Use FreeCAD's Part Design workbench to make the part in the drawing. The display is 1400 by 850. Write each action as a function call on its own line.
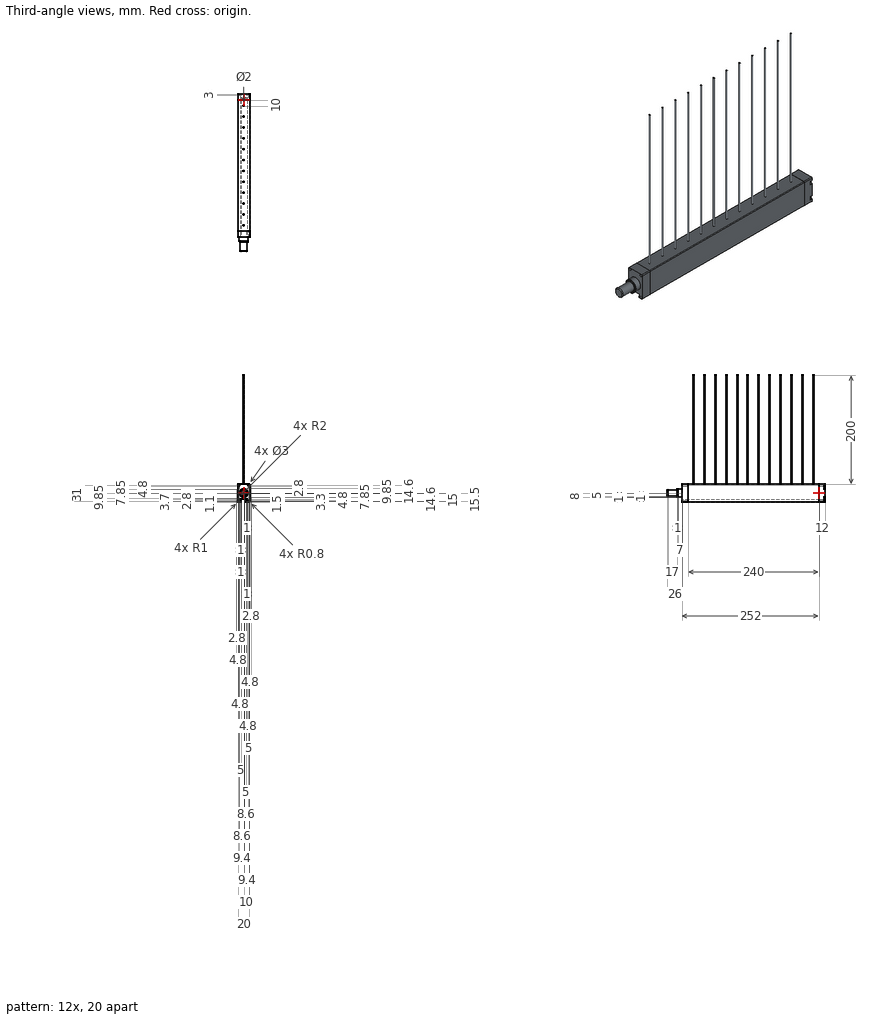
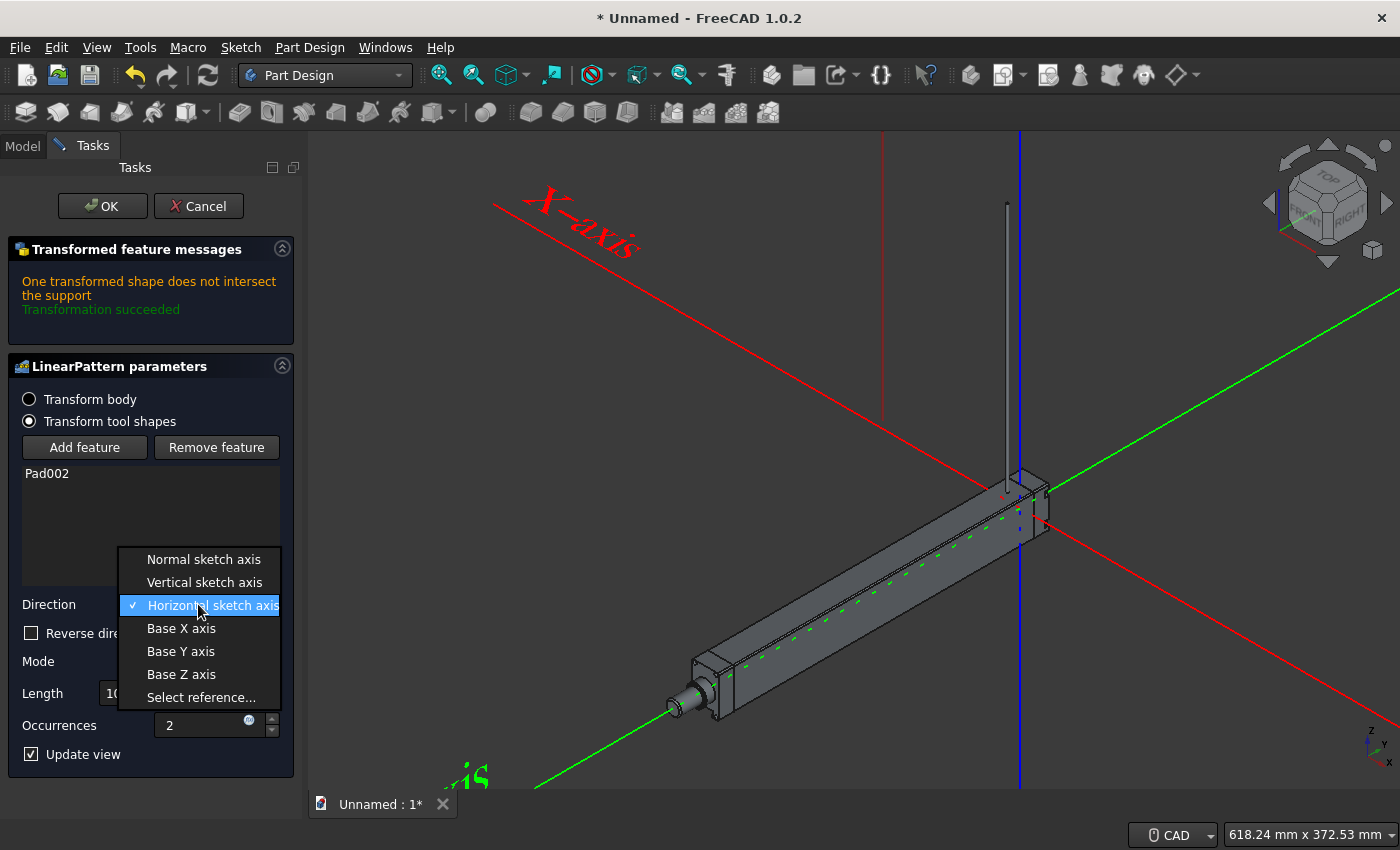
click(198, 652)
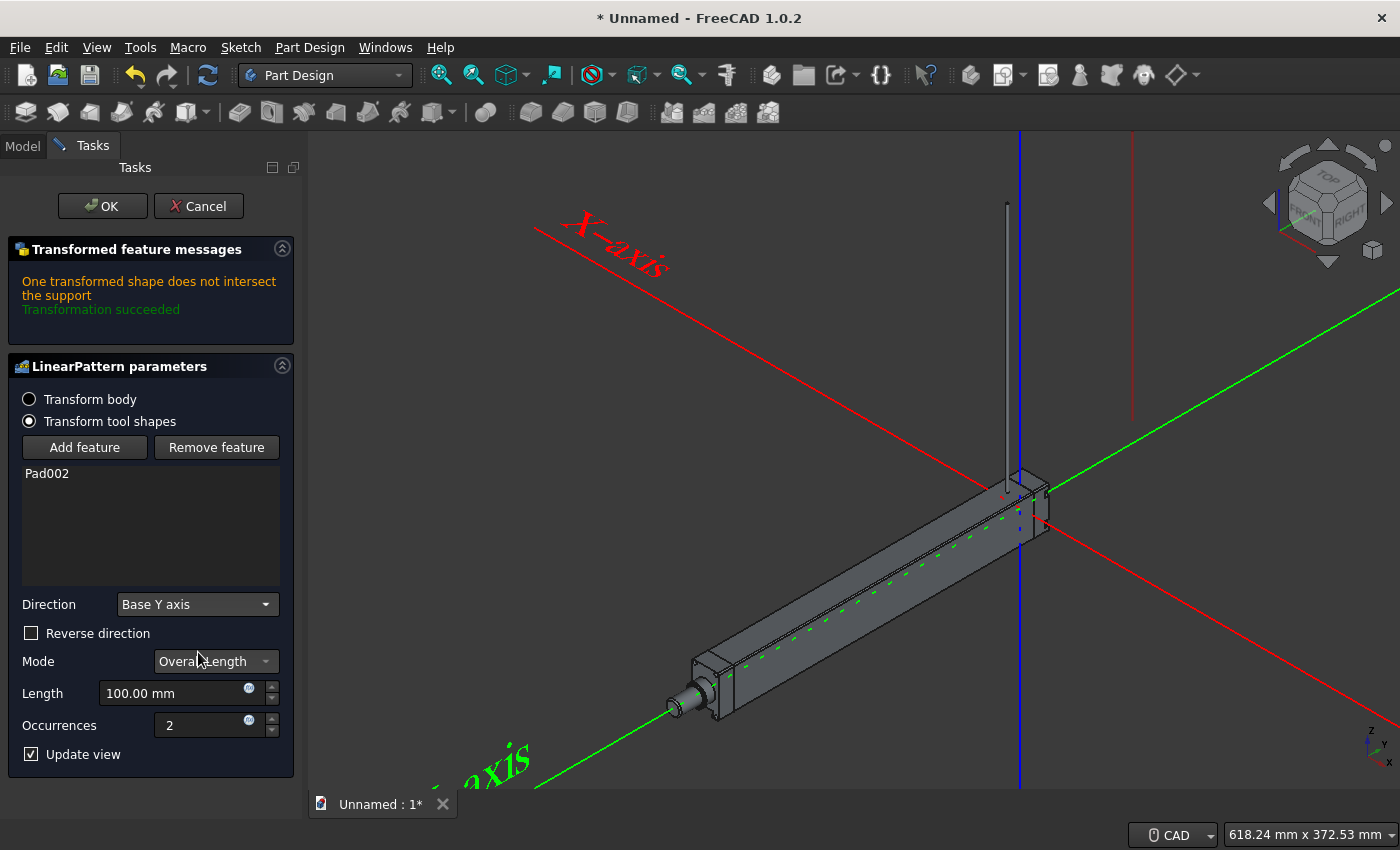
click(217, 662)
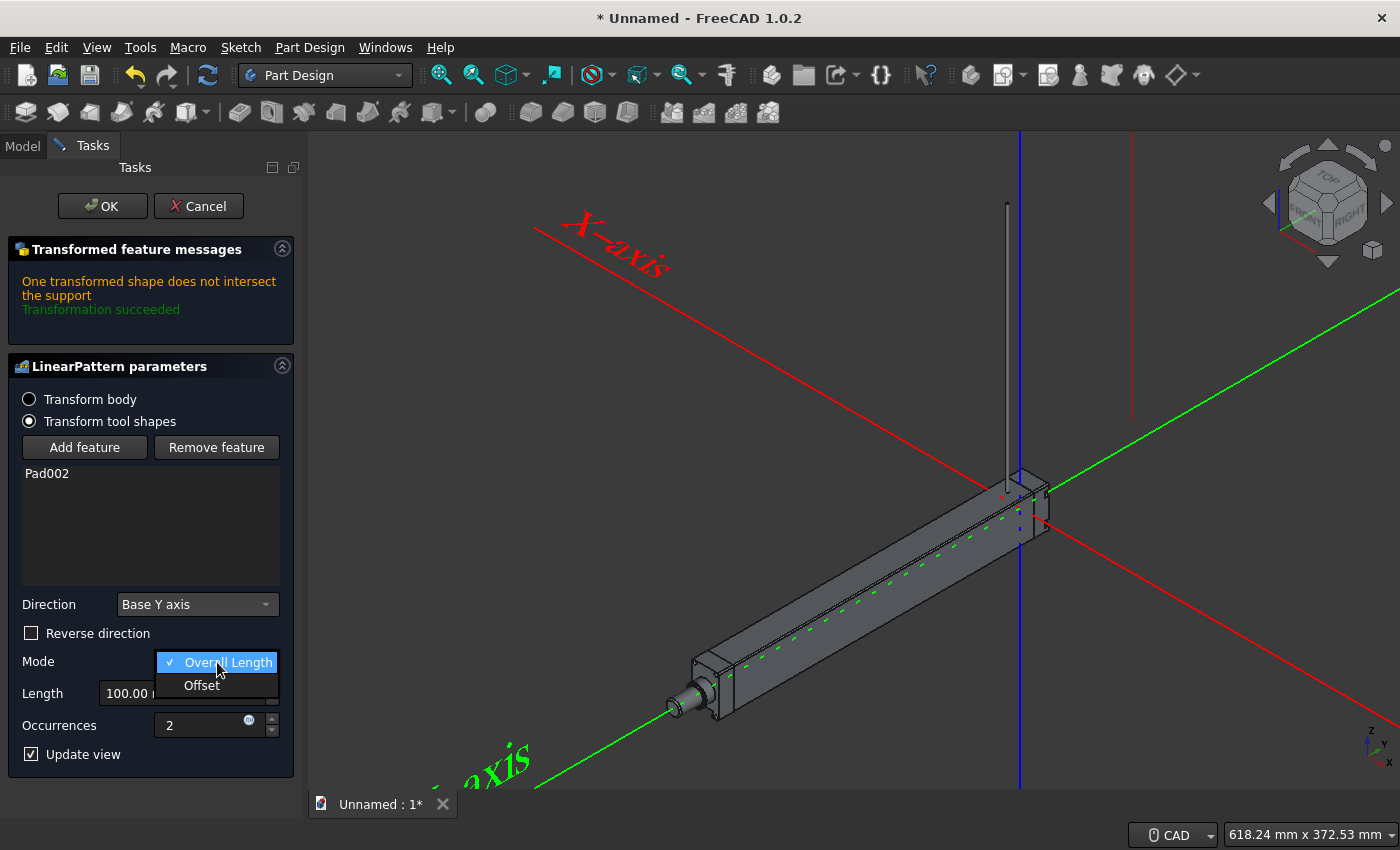
click(216, 686)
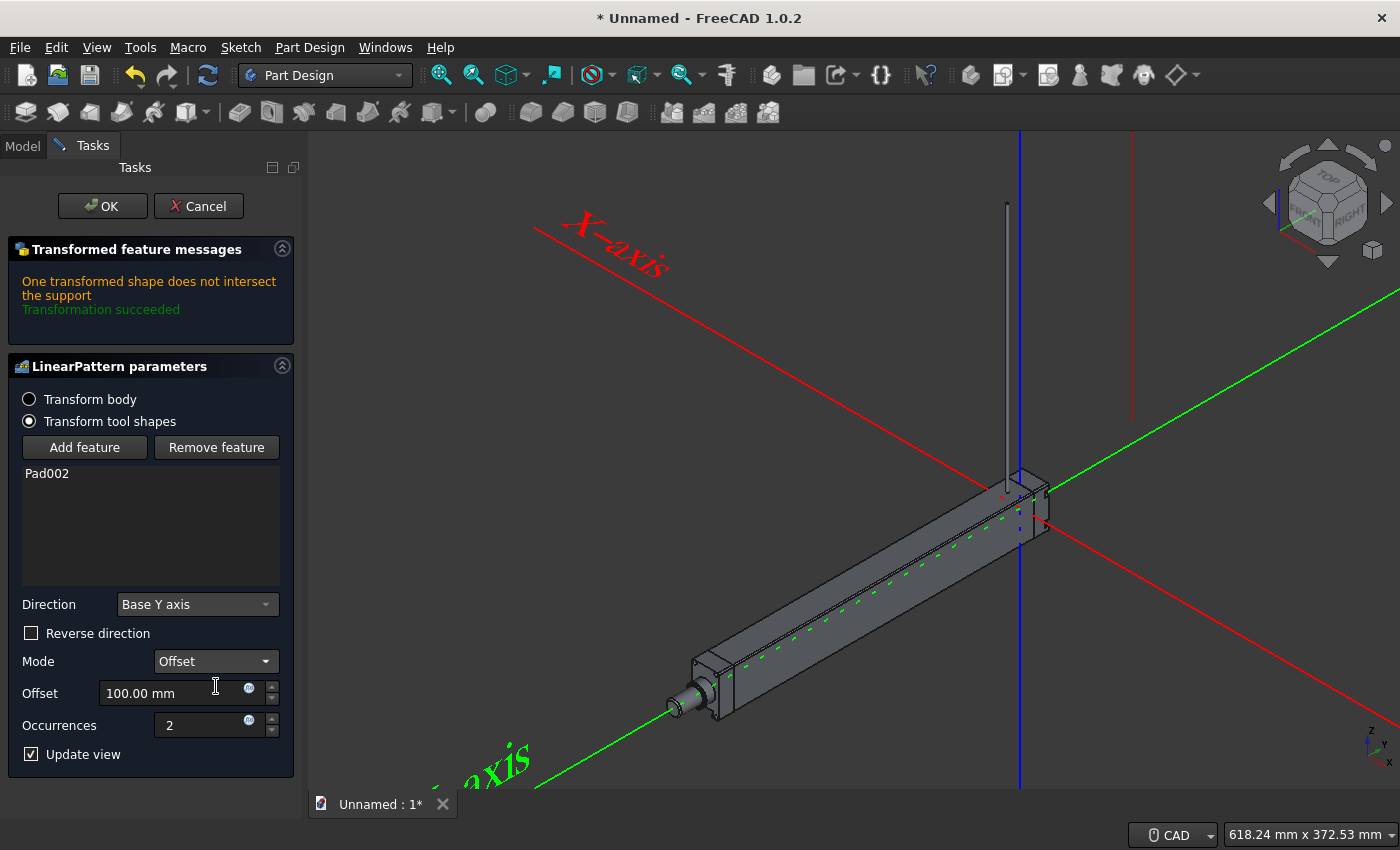
triple_click(182, 693)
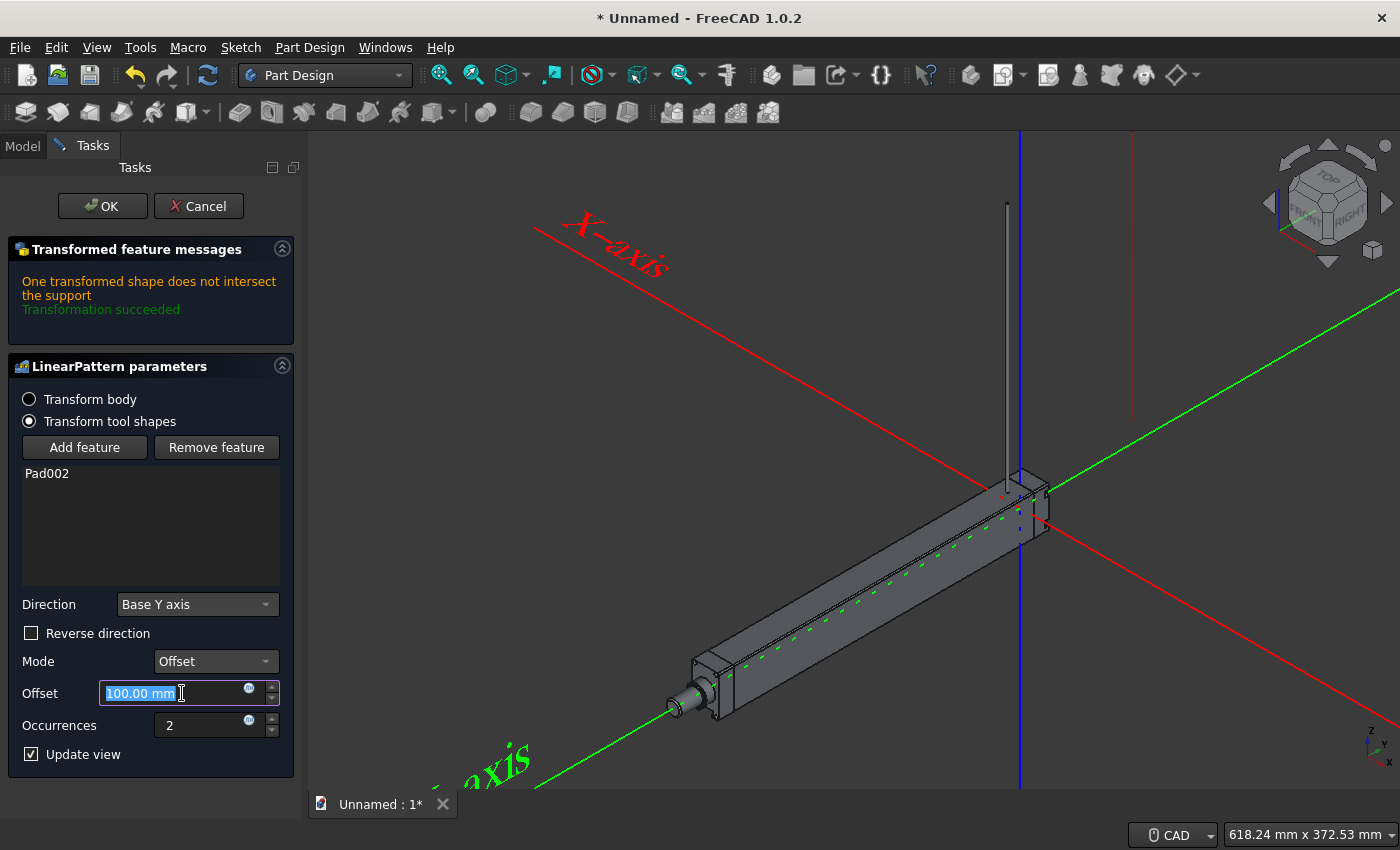
text(20)
key(Tab)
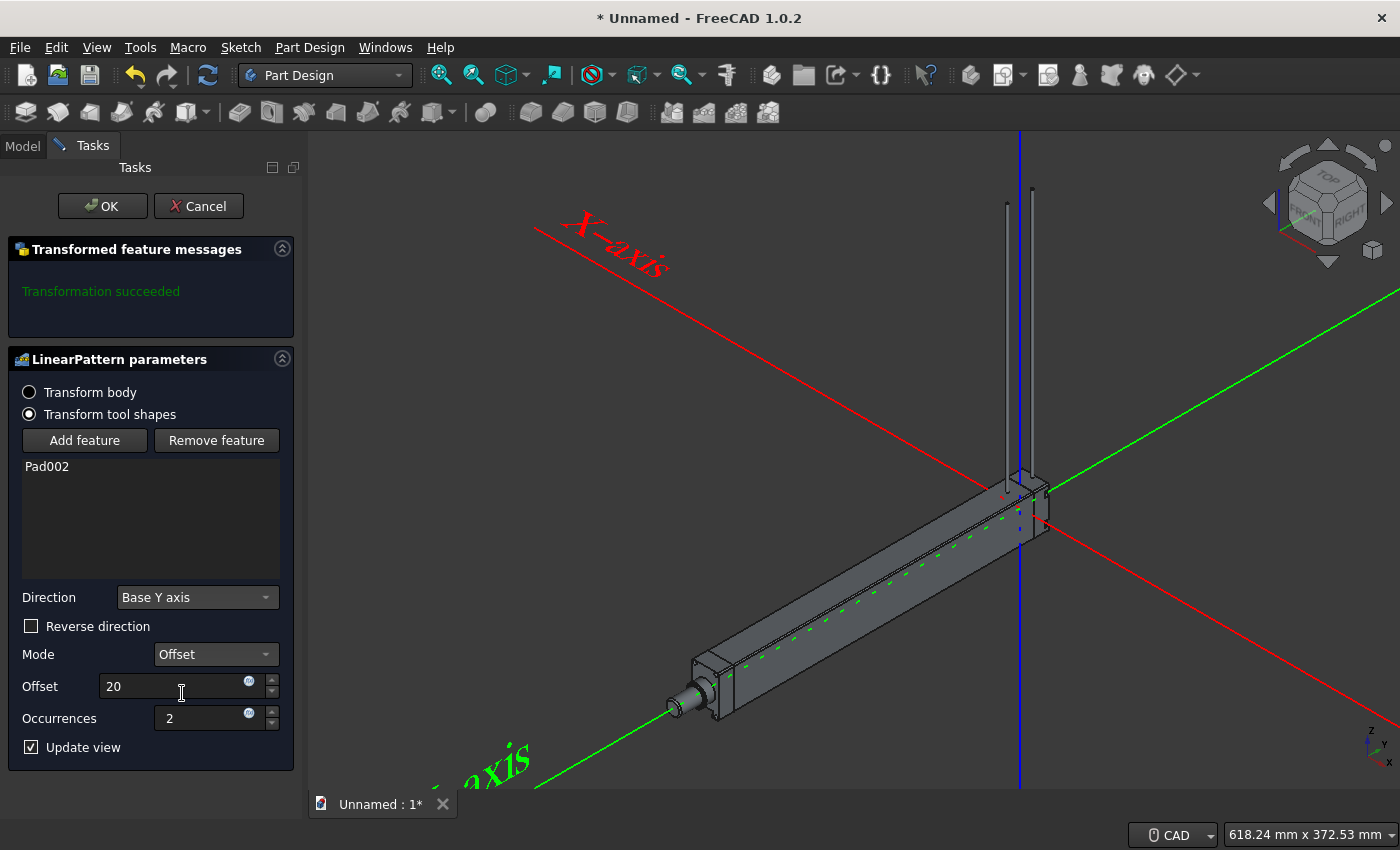
triple_click(209, 718)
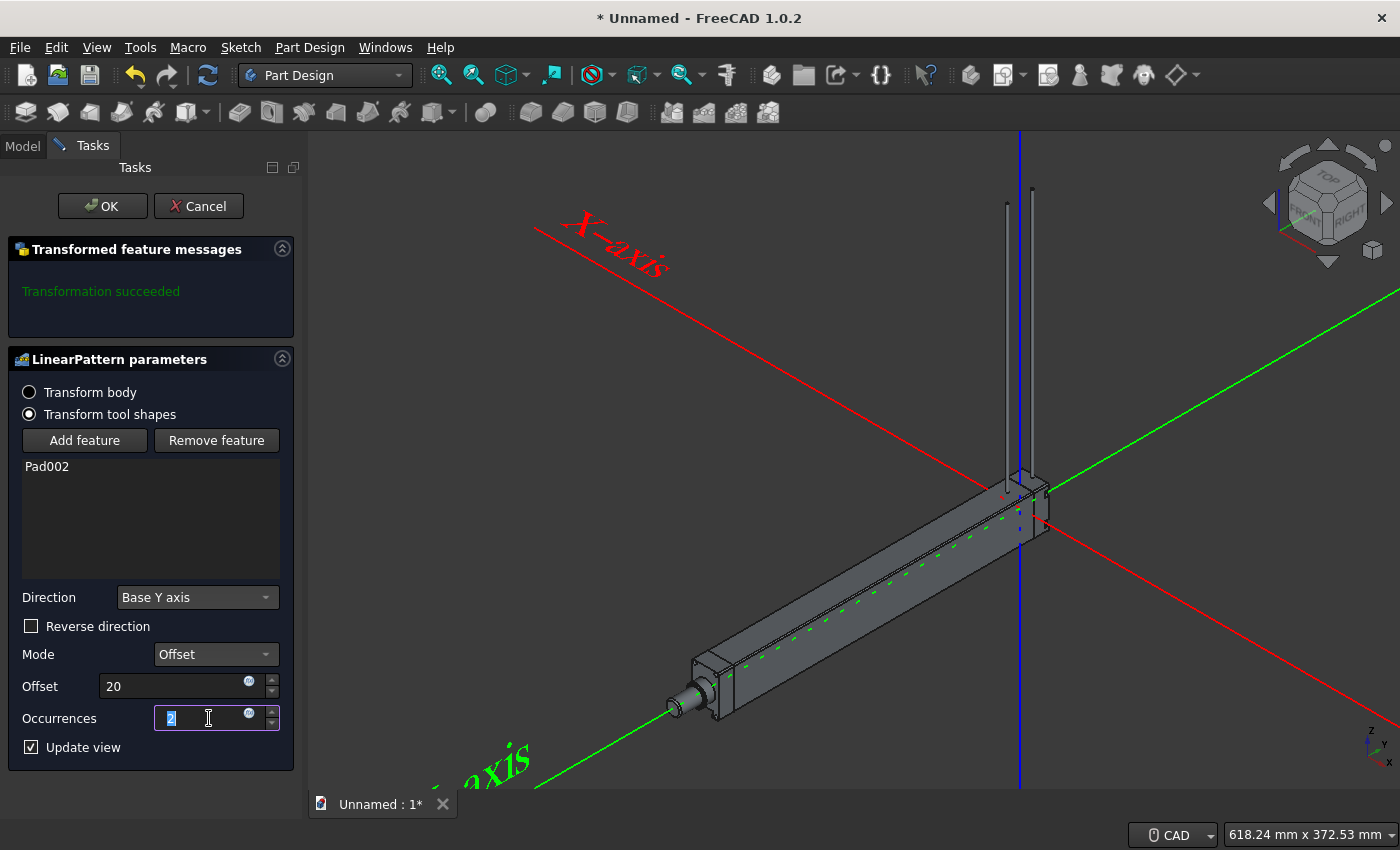
text(12)
key(Tab)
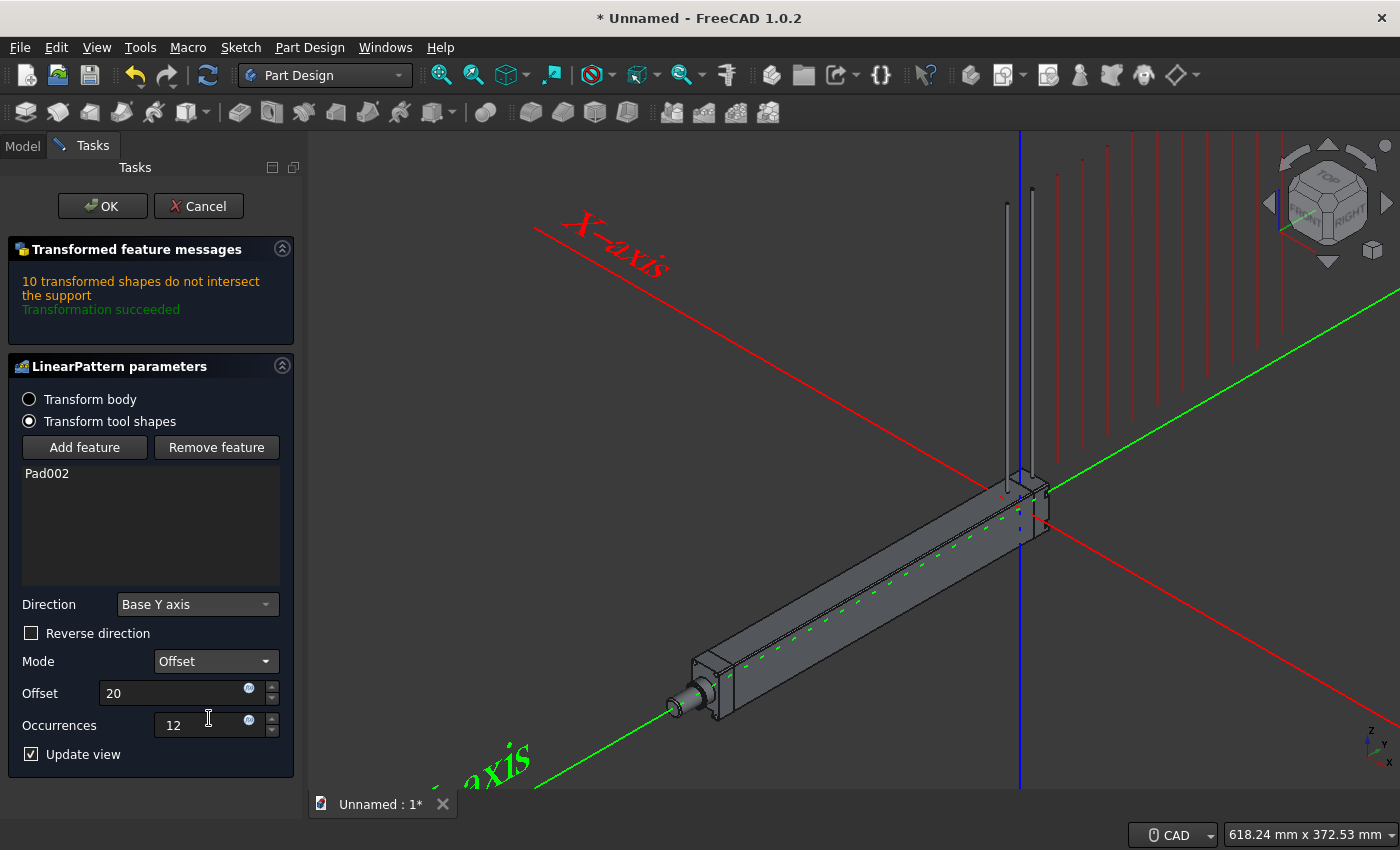
click(30, 633)